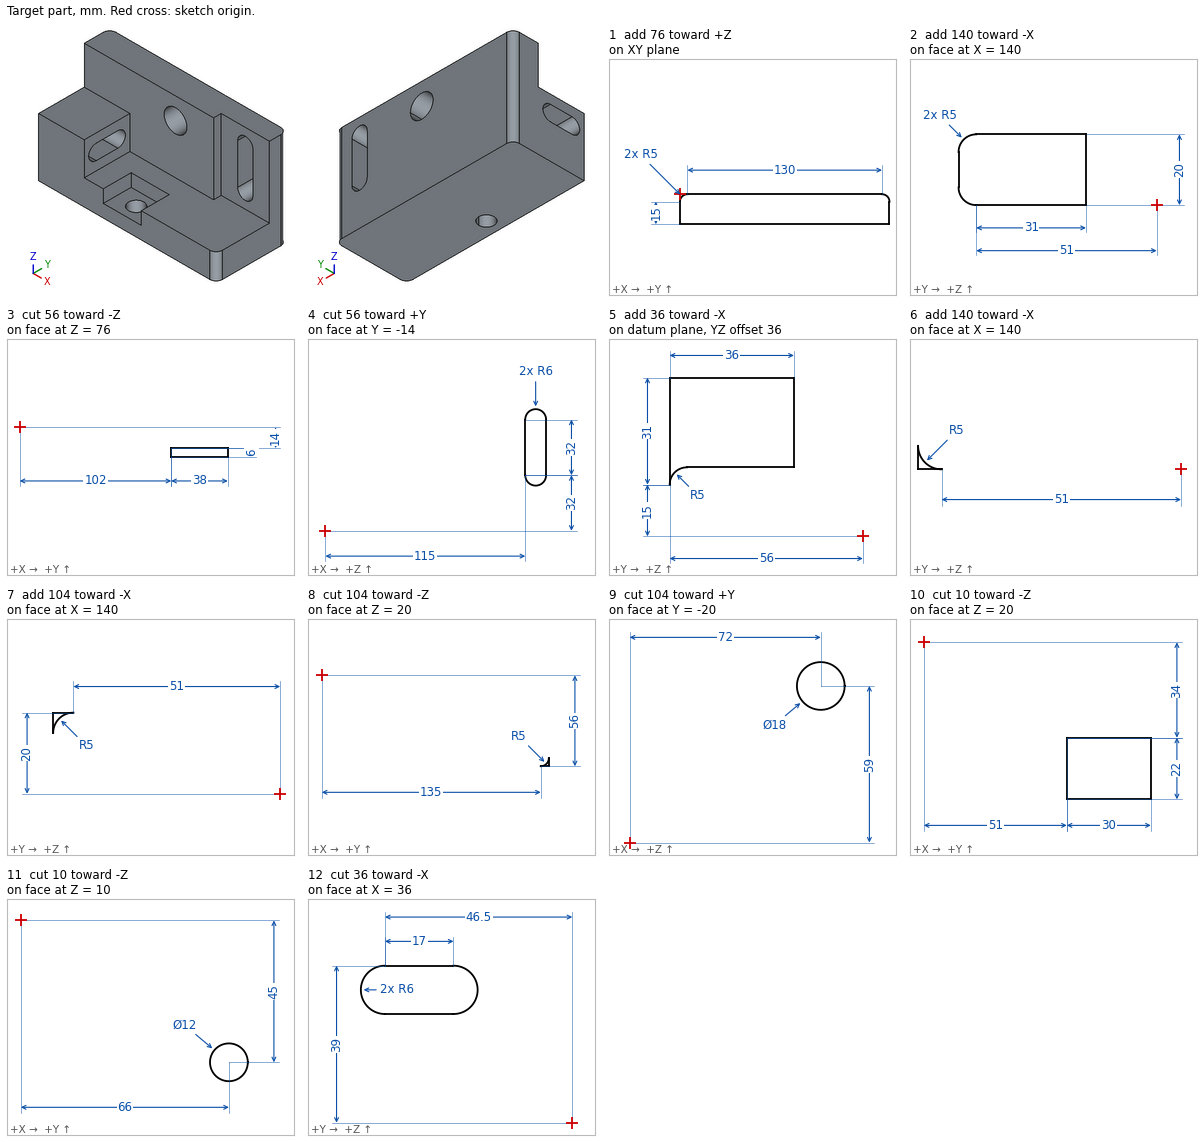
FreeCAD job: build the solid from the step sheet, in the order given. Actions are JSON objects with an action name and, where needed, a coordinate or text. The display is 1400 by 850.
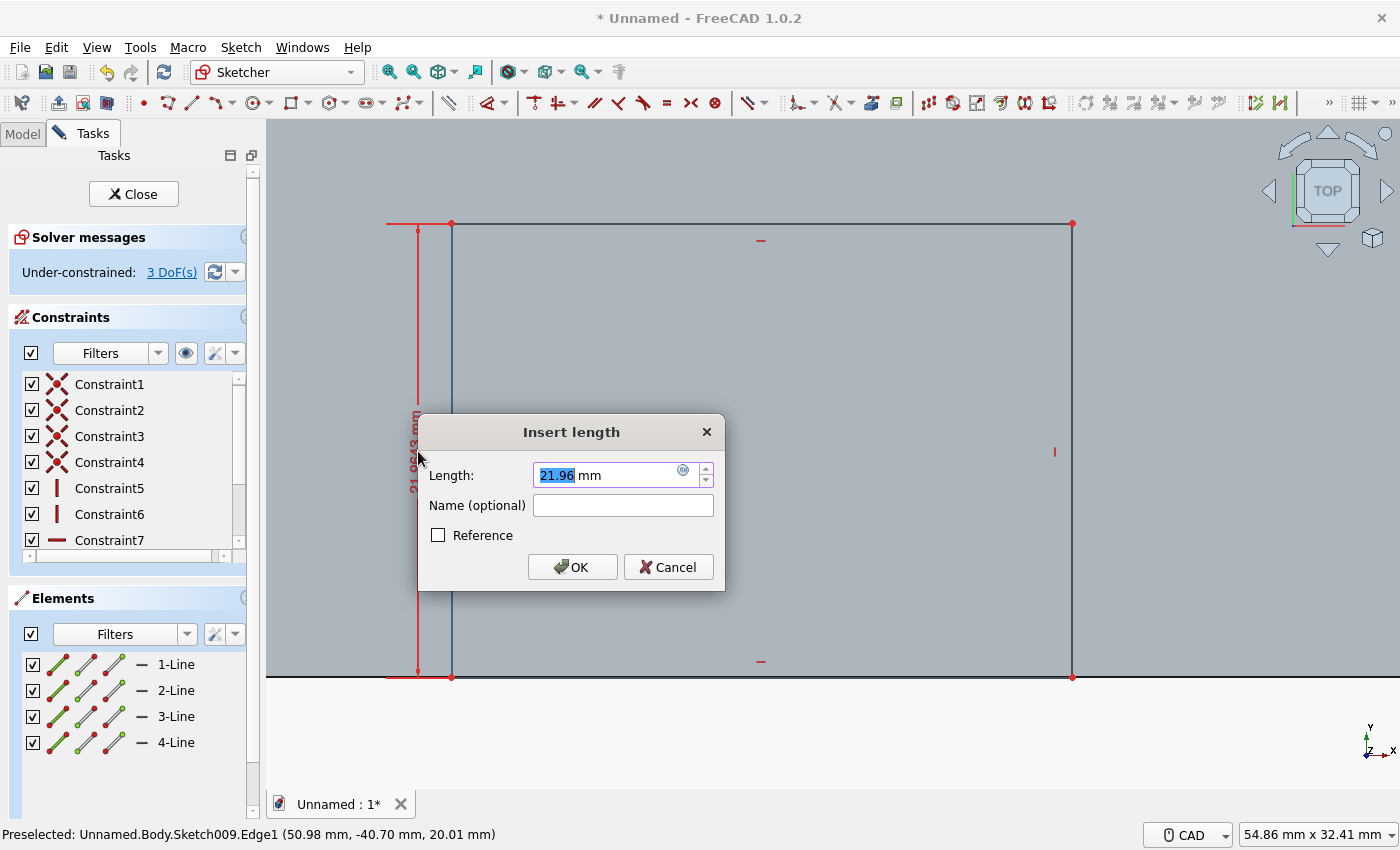
{"action": "type", "text": "22"}
{"action": "key", "text": "Return"}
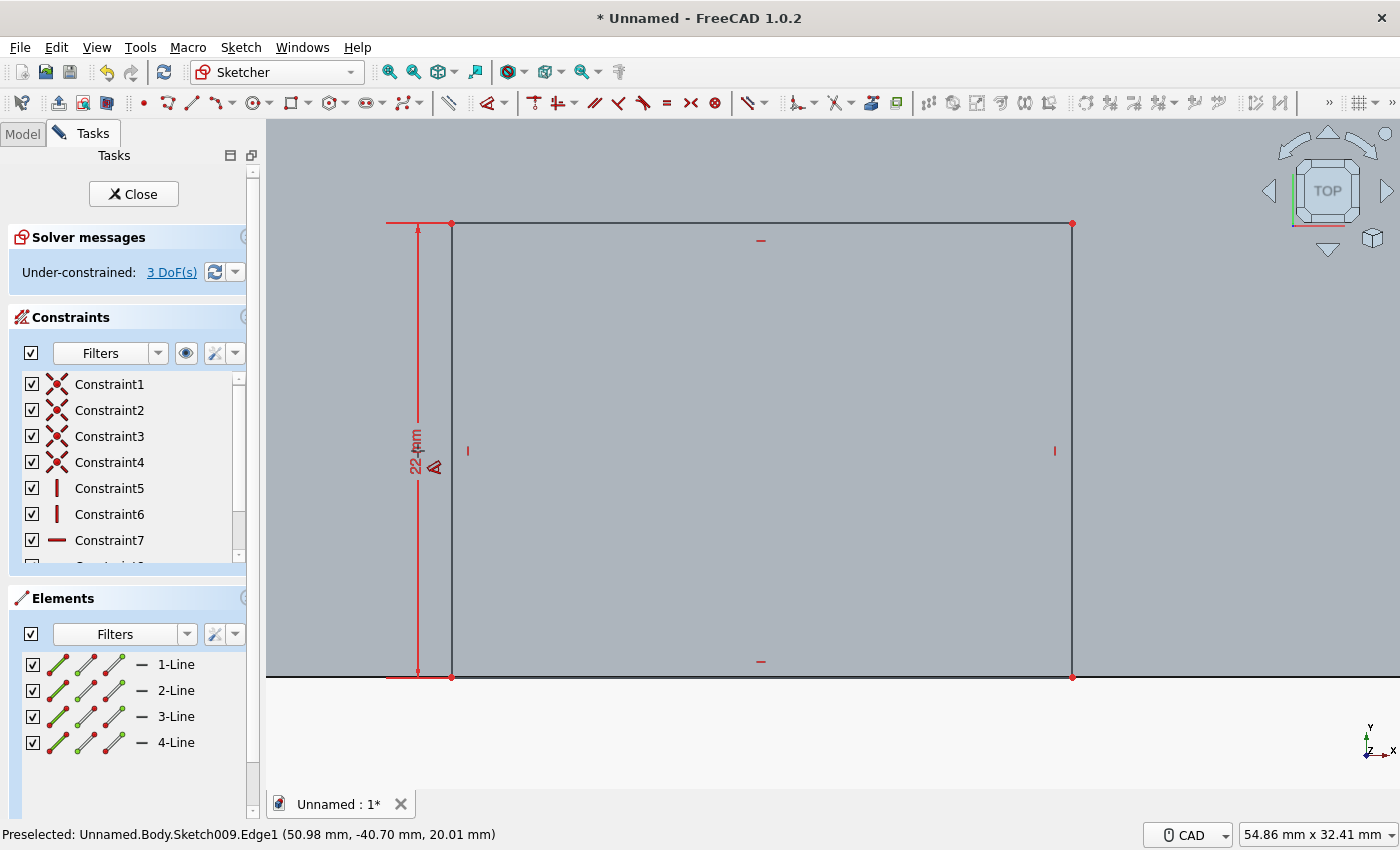
{"action": "left_click", "coordinate": [638, 678]}
{"action": "left_click", "coordinate": [762, 712]}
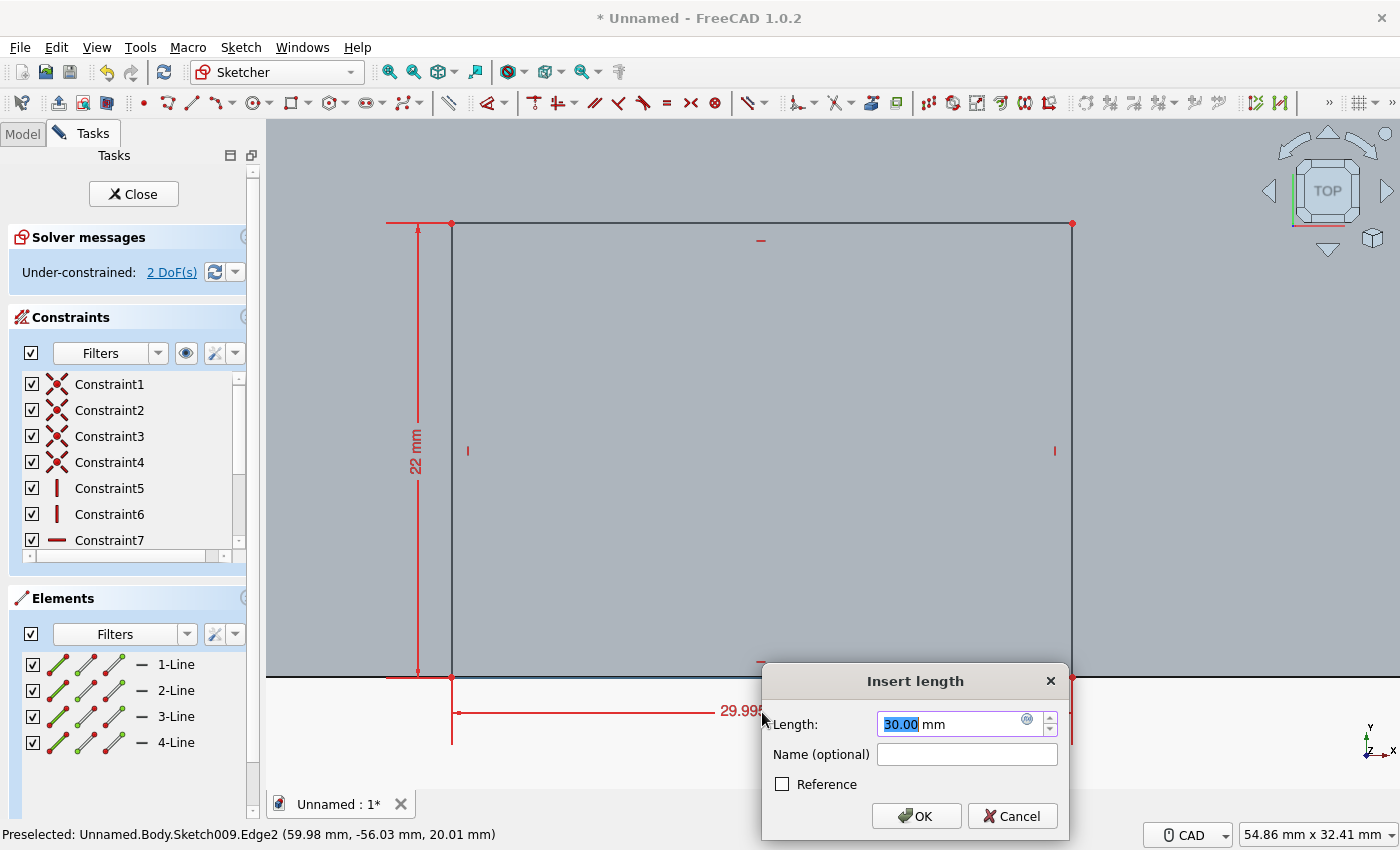
{"action": "type", "text": "30"}
{"action": "key", "text": "Return"}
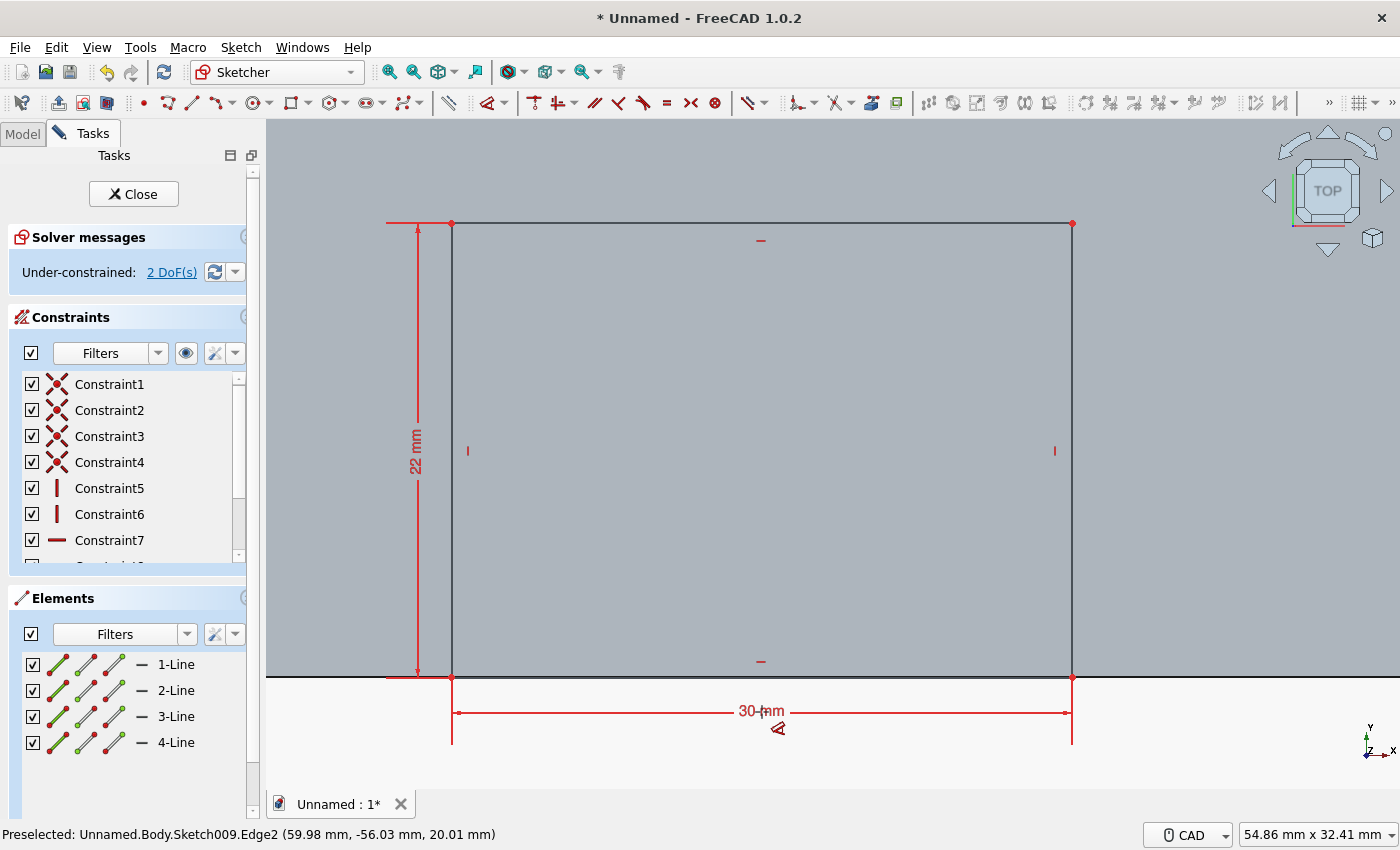
{"action": "left_click", "coordinate": [452, 223]}
{"action": "left_click", "coordinate": [373, 257]}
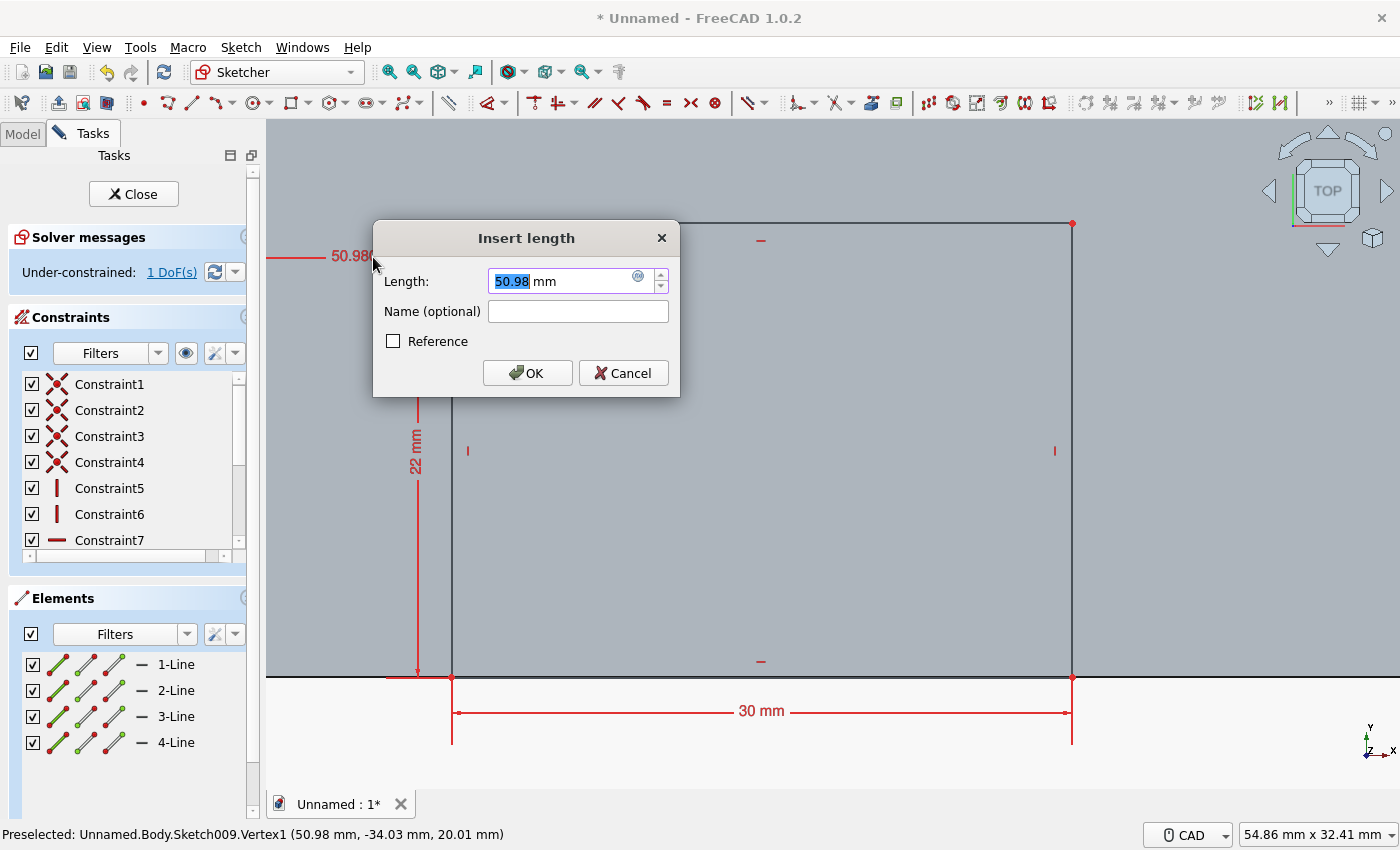
{"action": "type", "text": "51"}
{"action": "key", "text": "Return"}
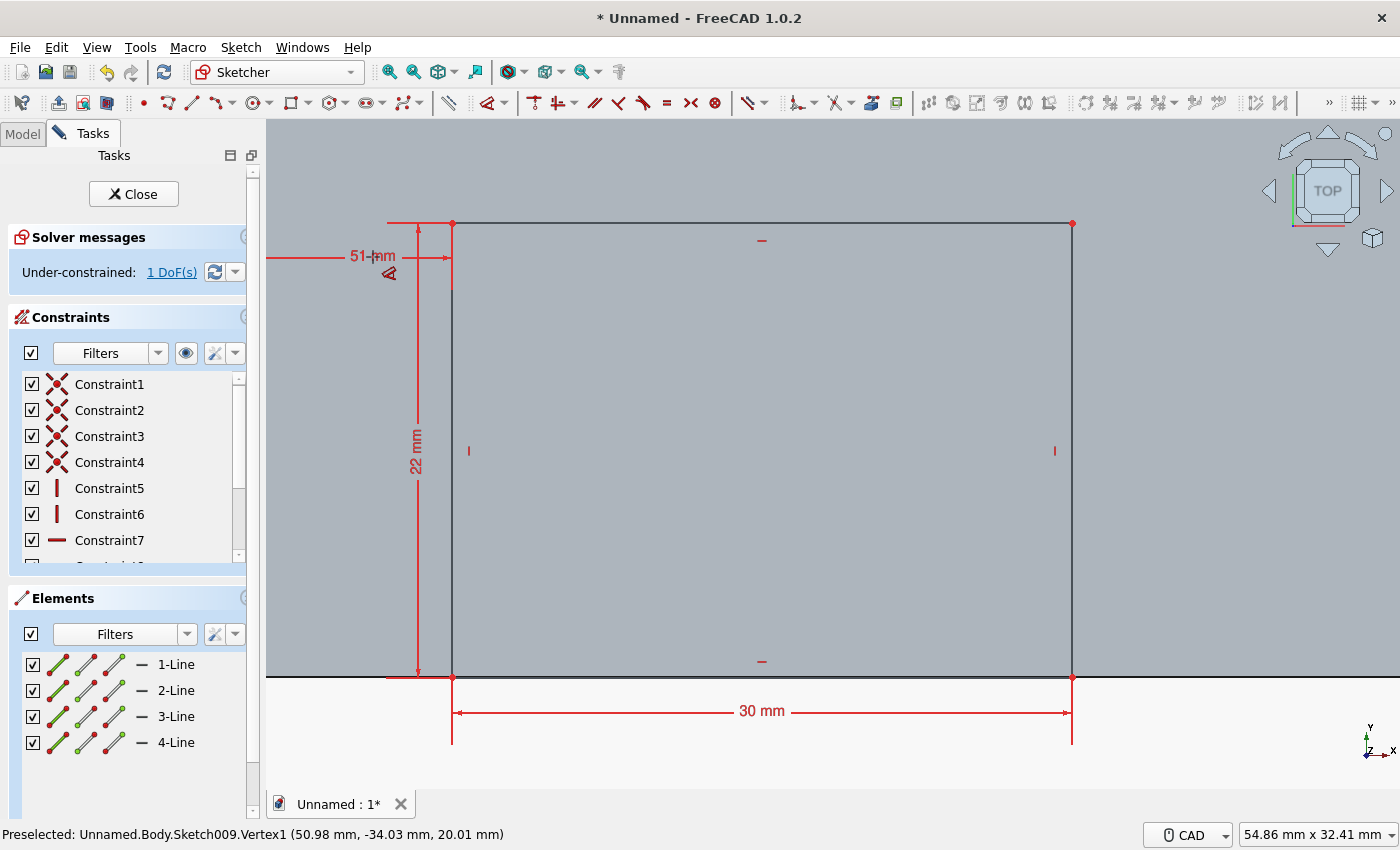
{"action": "left_click", "coordinate": [452, 223]}
{"action": "left_click", "coordinate": [486, 185]}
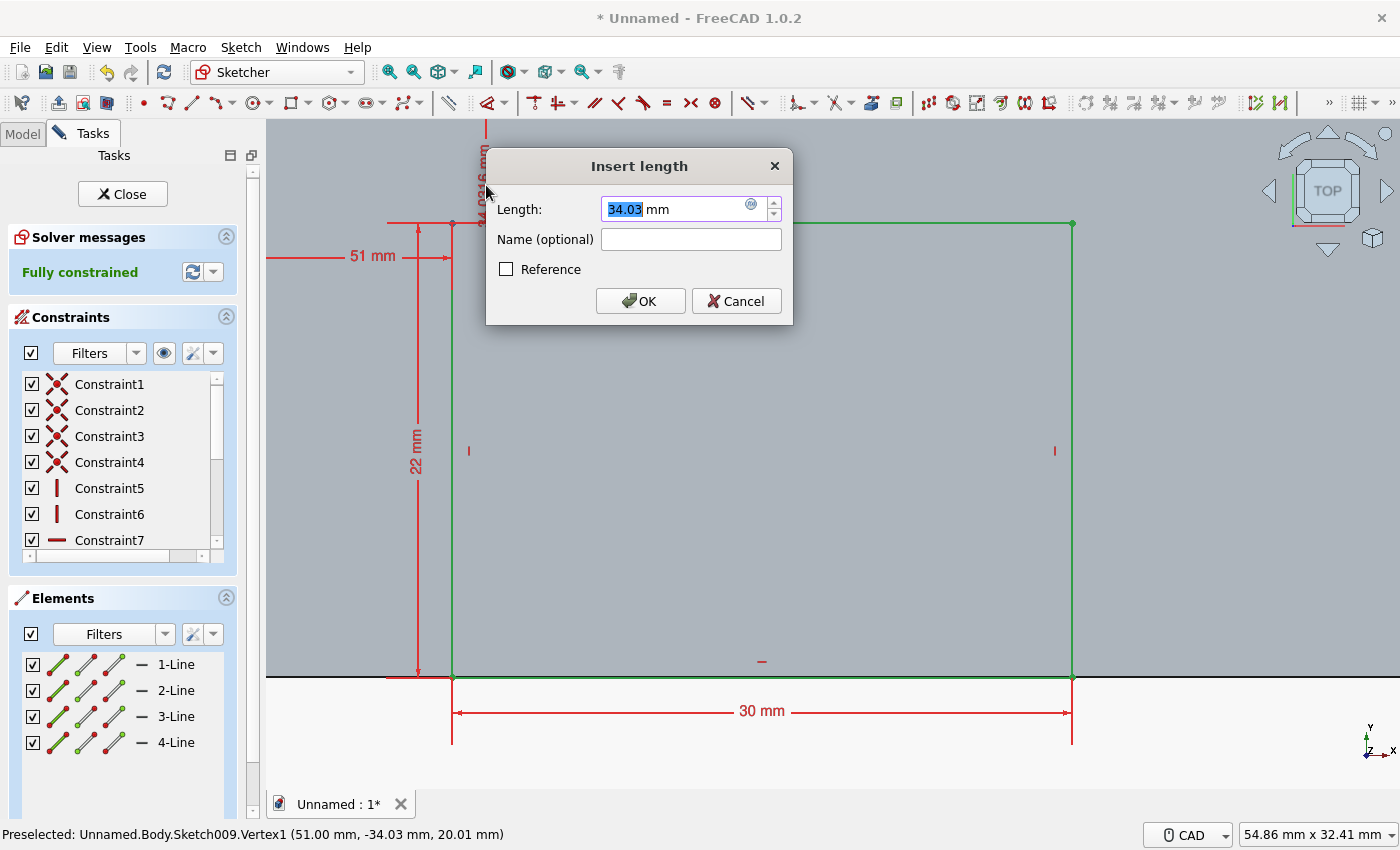
{"action": "type", "text": "34"}
{"action": "key", "text": "Return"}
{"action": "key", "text": "Escape"}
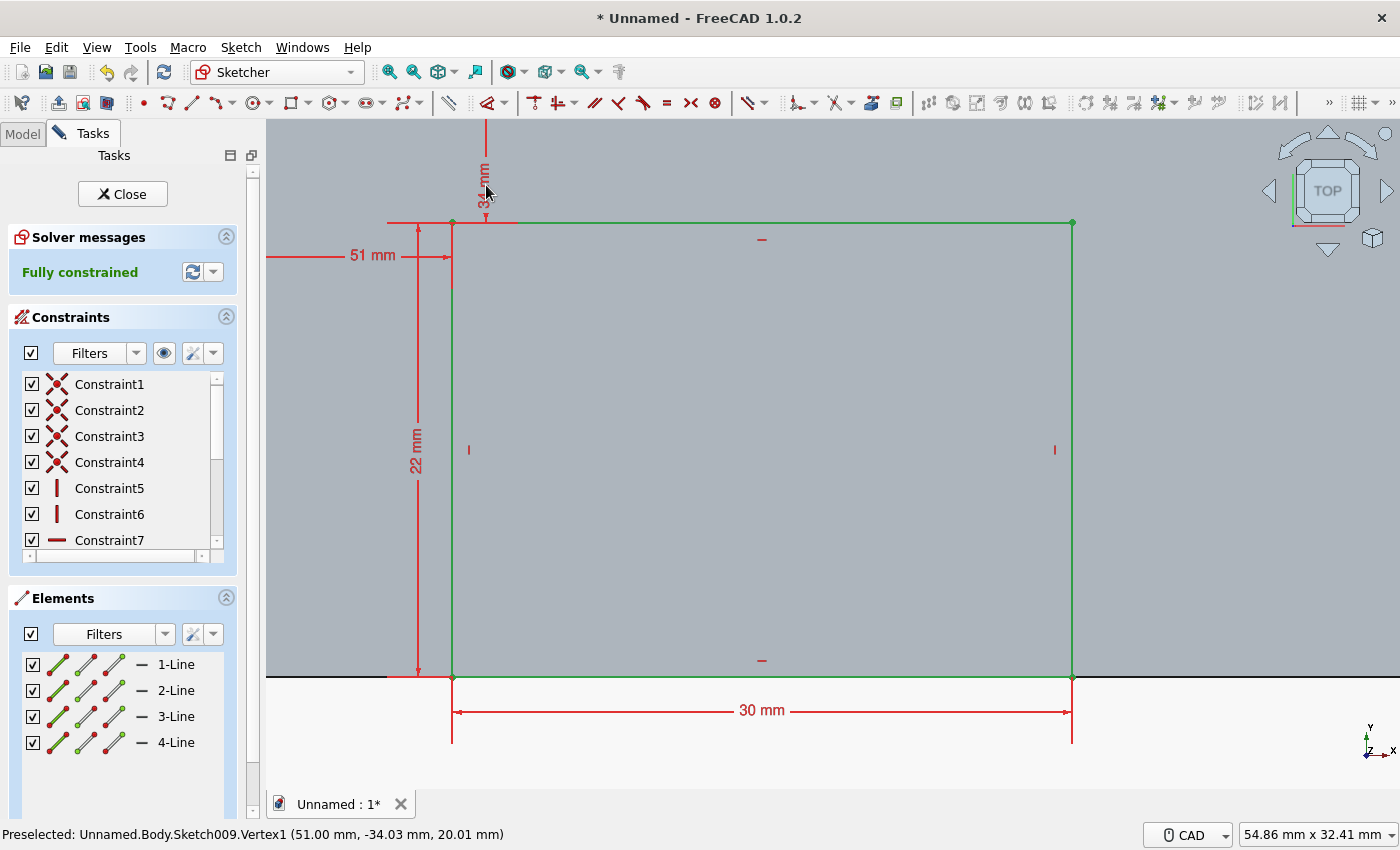
{"action": "left_click", "coordinate": [123, 194]}